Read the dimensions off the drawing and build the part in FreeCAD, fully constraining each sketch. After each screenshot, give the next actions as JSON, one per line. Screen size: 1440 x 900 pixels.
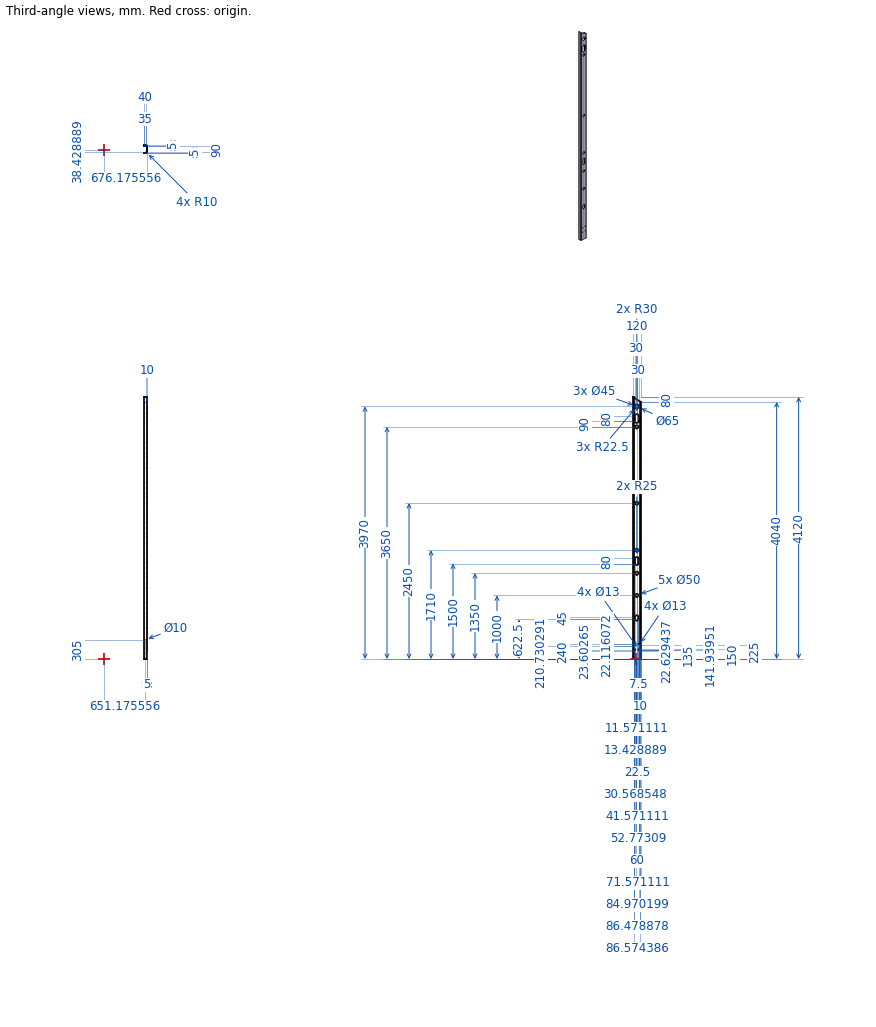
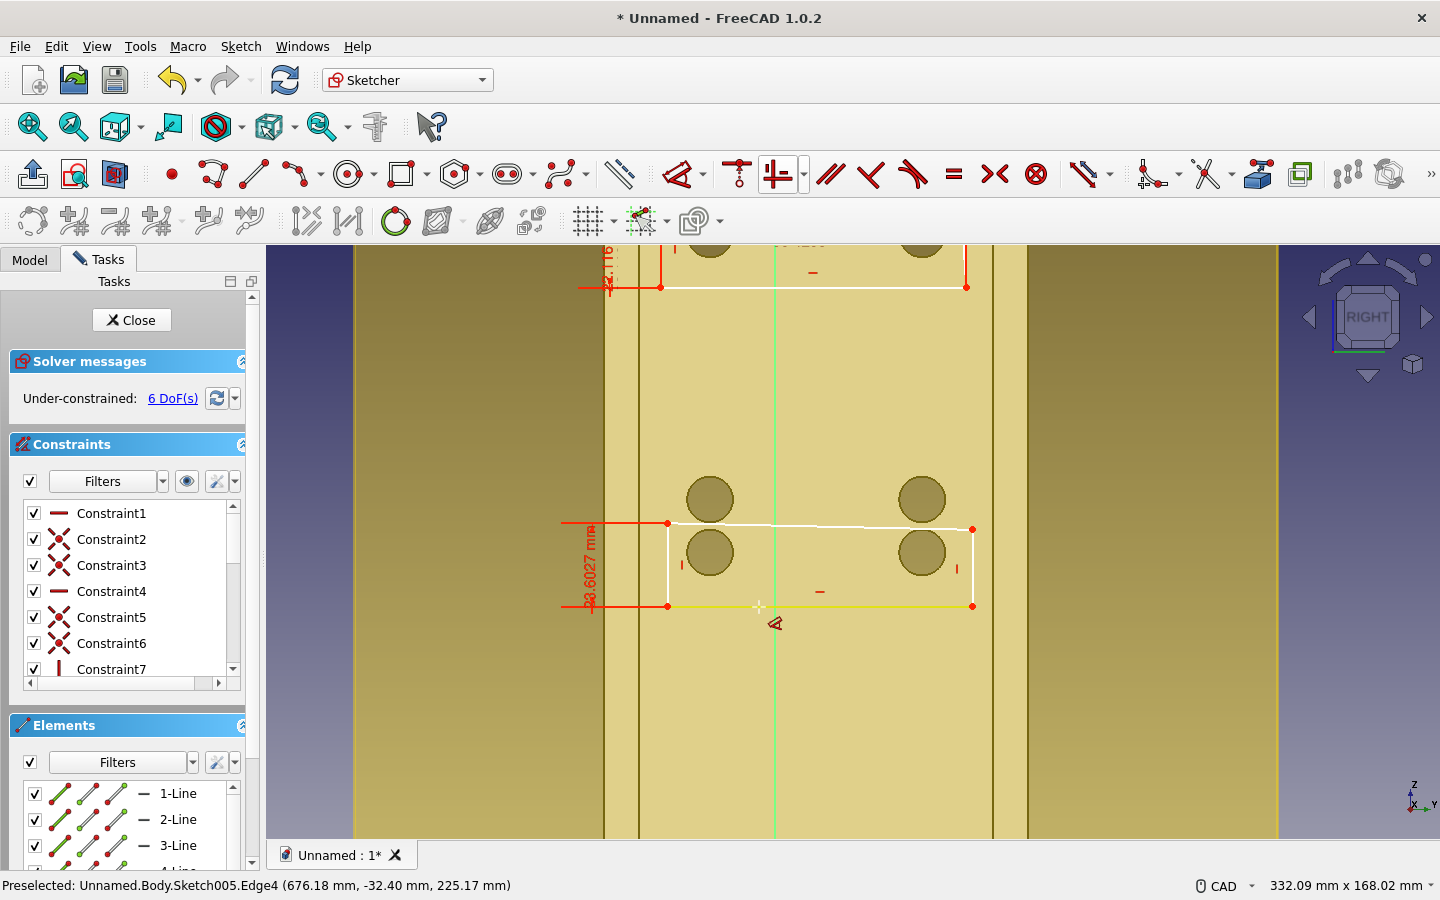
{"action": "left_click", "coordinate": [759, 607]}
{"action": "left_click", "coordinate": [820, 573]}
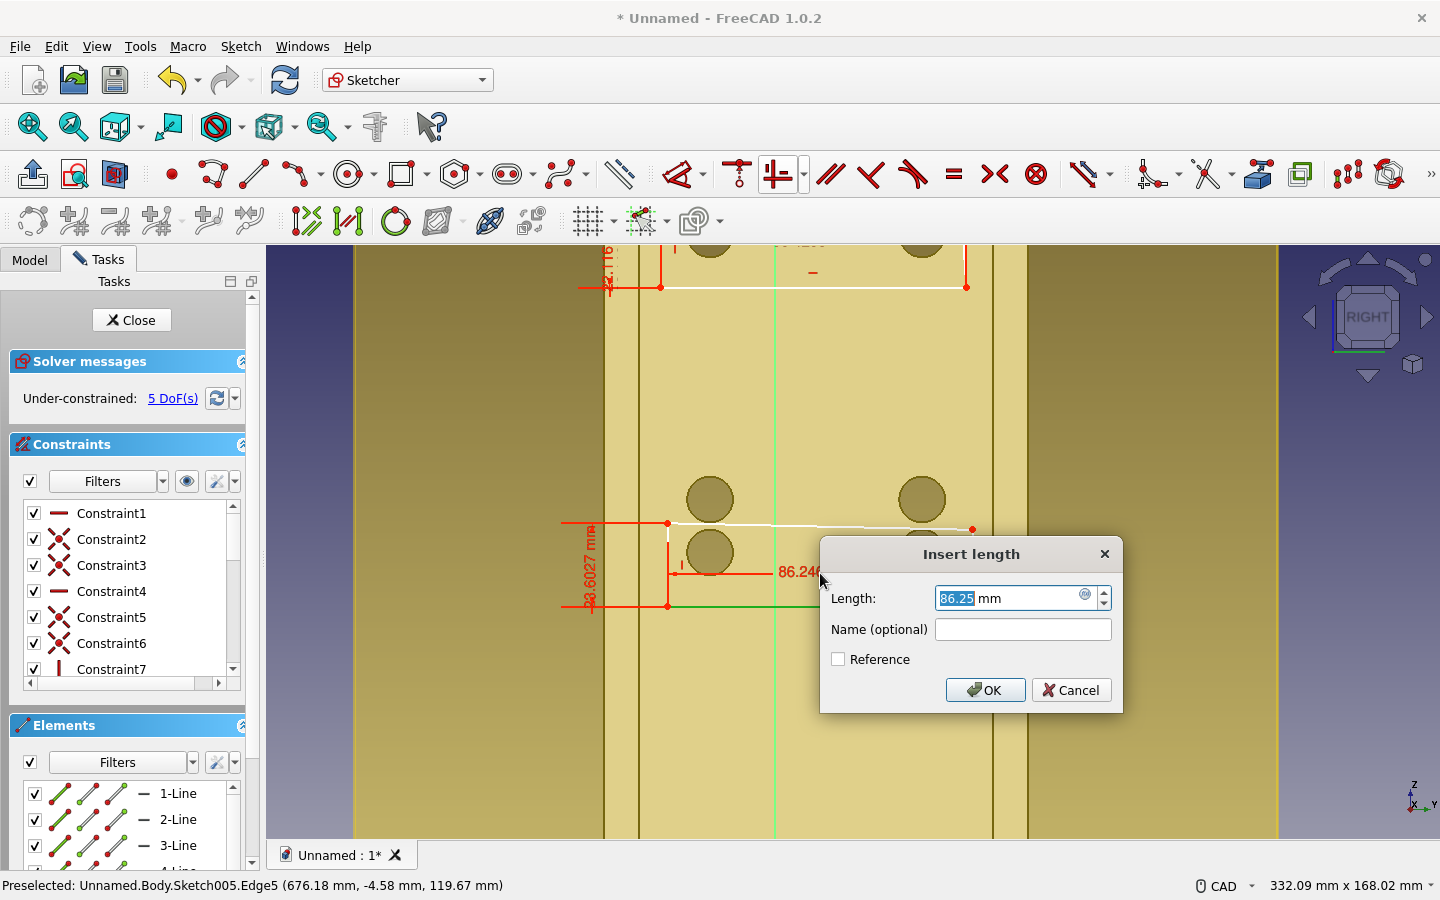
{"action": "type", "text": "86.574386"}
{"action": "key", "text": "Return"}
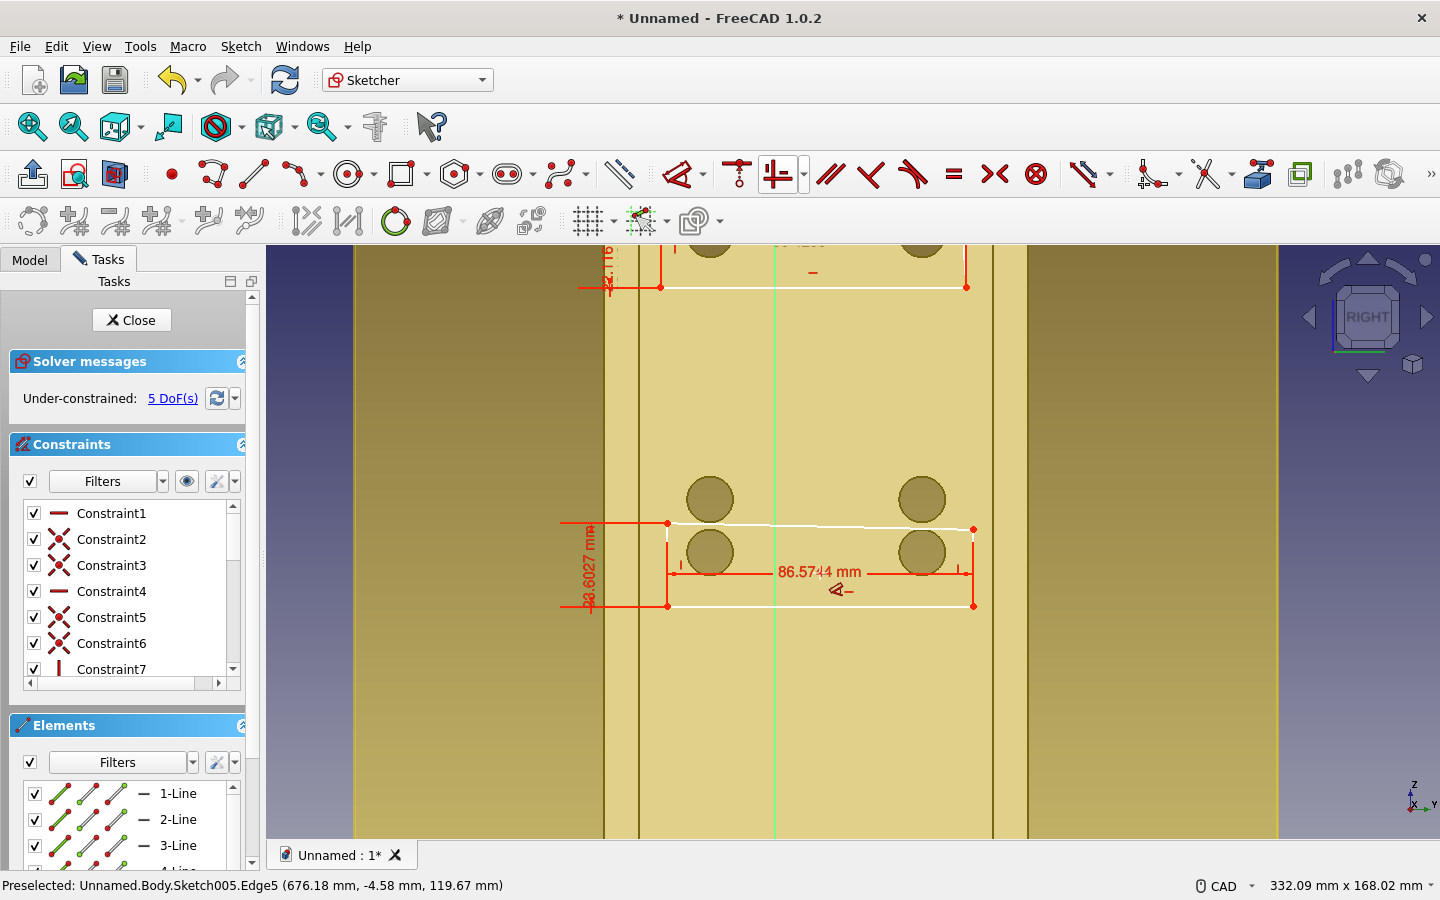
{"action": "left_click", "coordinate": [973, 584]}
{"action": "left_click", "coordinate": [1007, 568]}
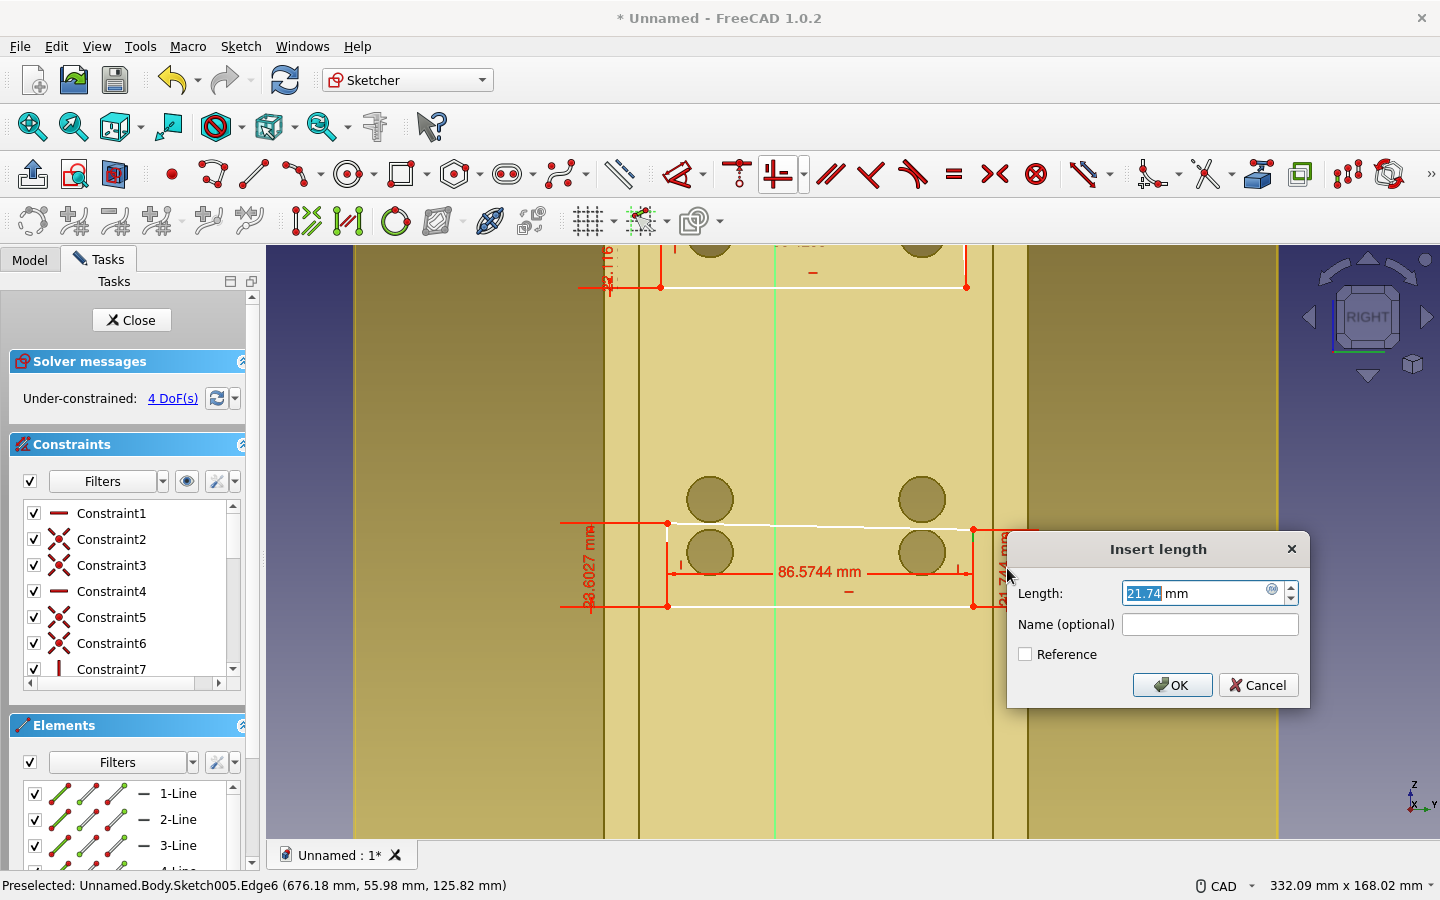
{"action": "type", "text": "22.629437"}
{"action": "key", "text": "Return"}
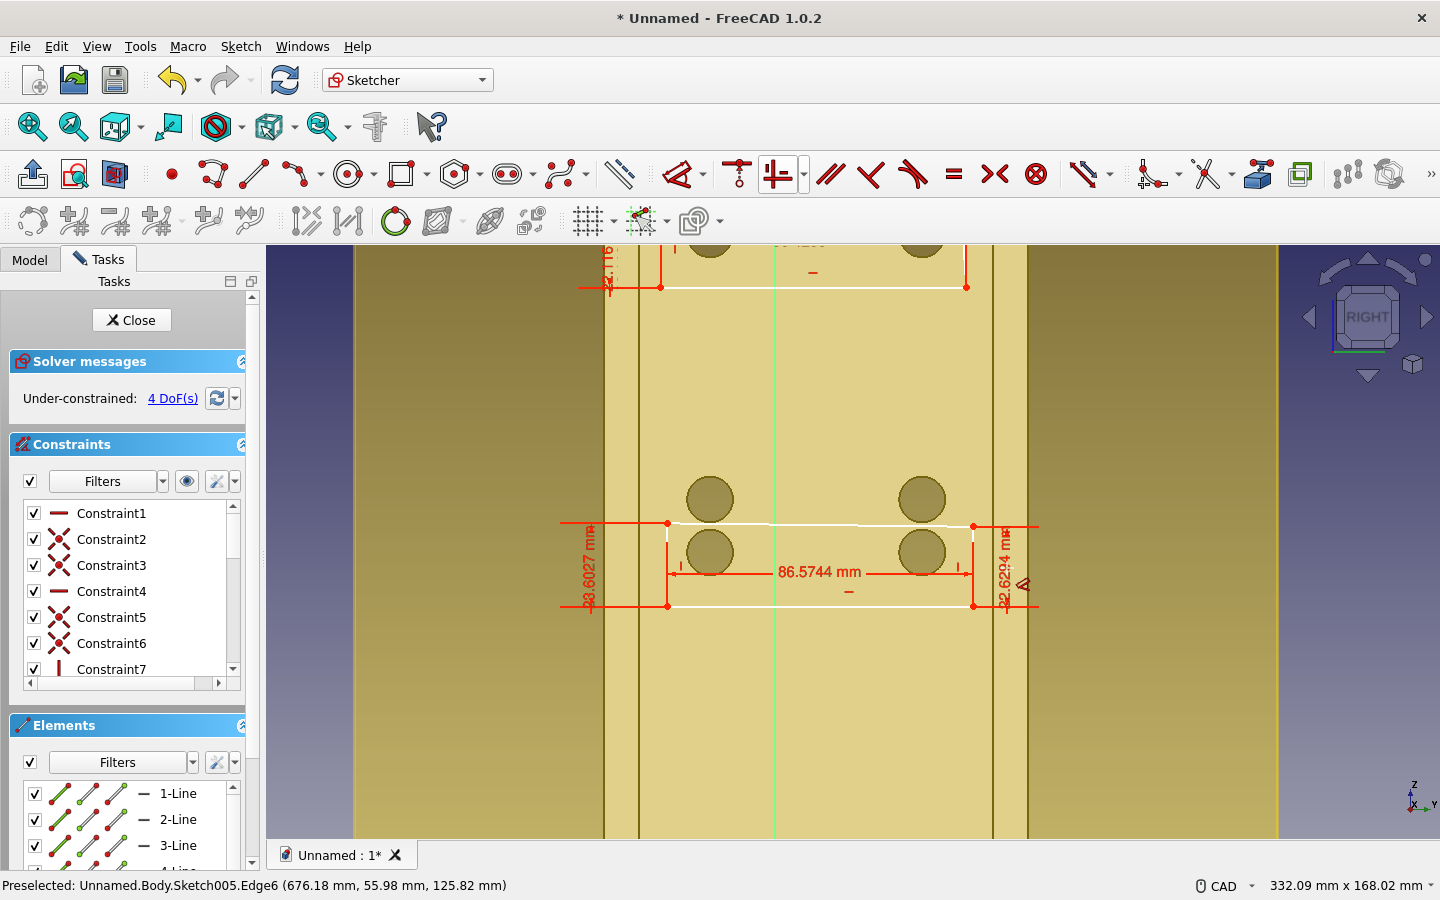
{"action": "scroll", "coordinate": [758, 480], "scroll_direction": "down", "scroll_amount": 4}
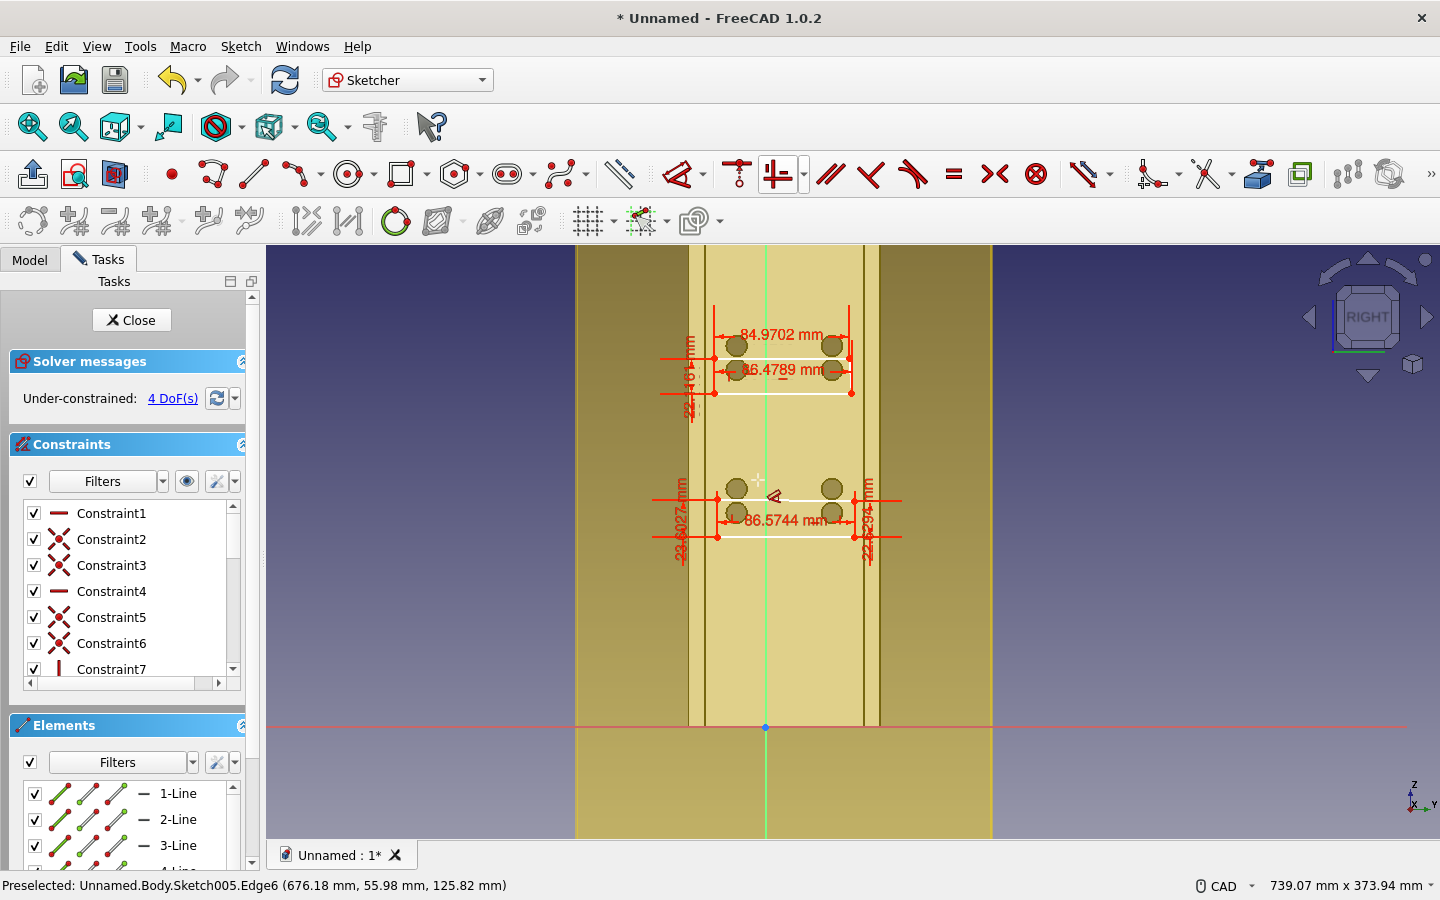
{"action": "left_click", "coordinate": [849, 359]}
{"action": "left_click", "coordinate": [808, 761]}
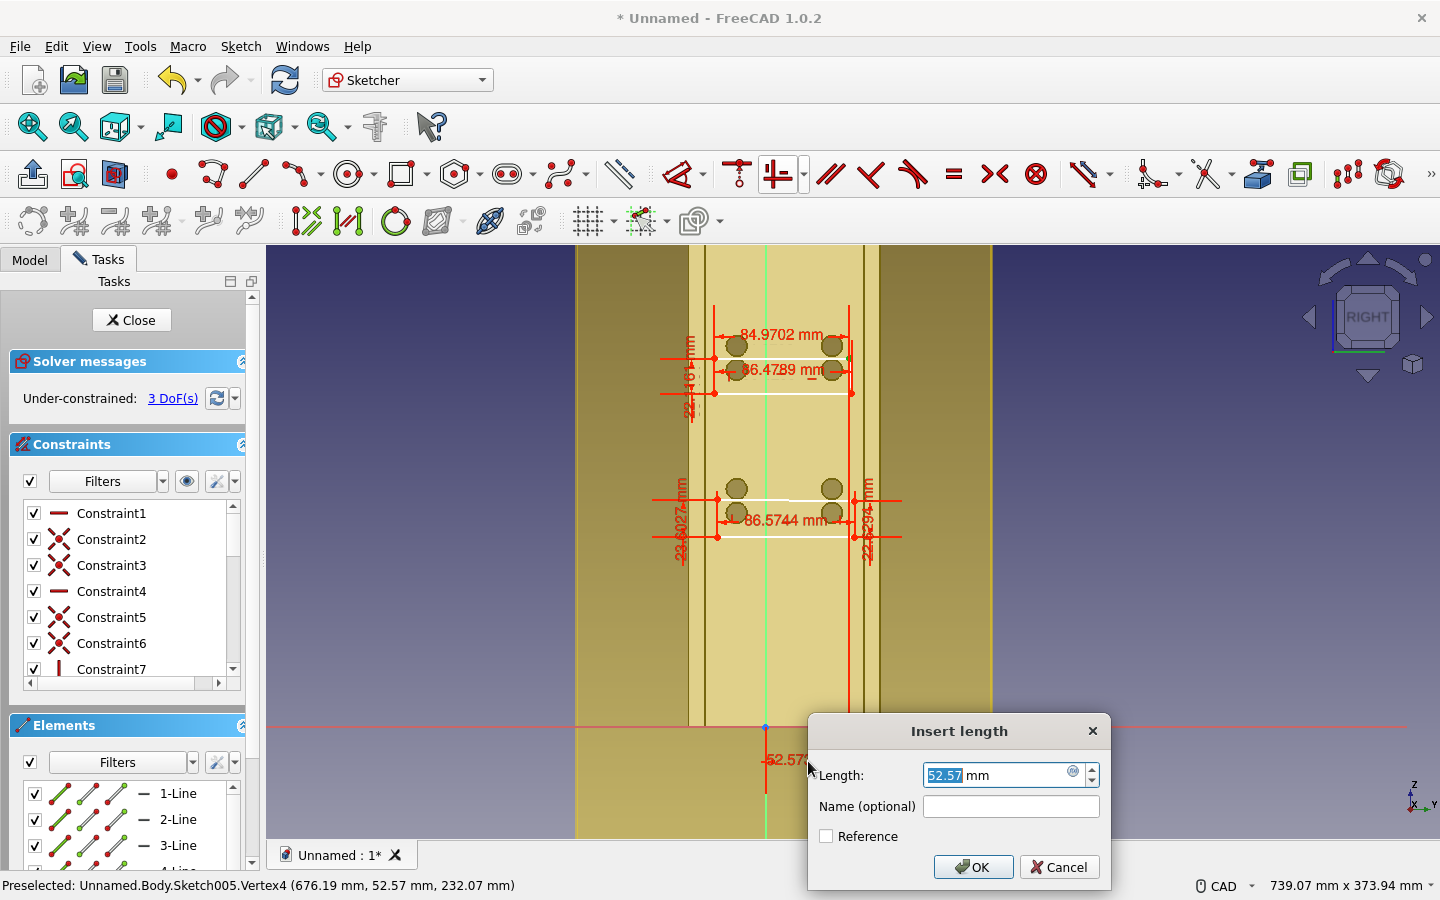
{"action": "type", "text": "52.77309"}
{"action": "key", "text": "Return"}